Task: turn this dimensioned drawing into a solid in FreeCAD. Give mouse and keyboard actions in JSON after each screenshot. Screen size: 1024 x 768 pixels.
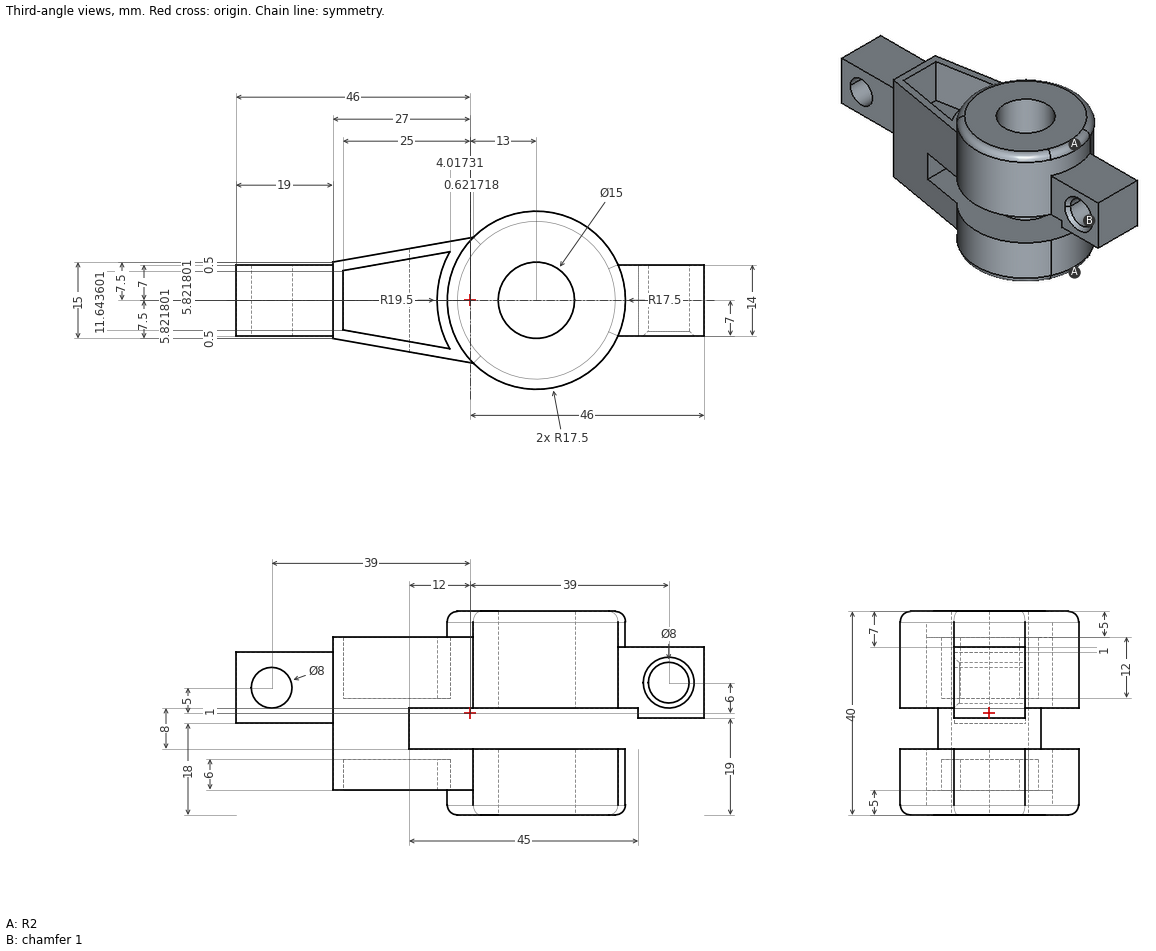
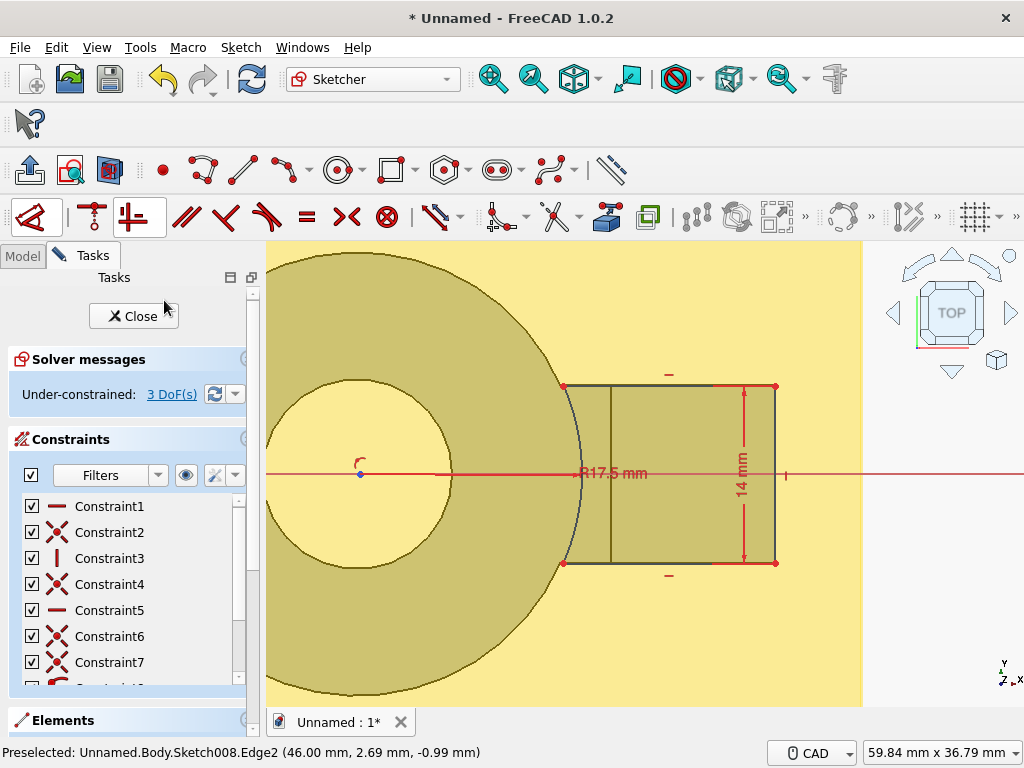
{"action": "left_click", "coordinate": [564, 386]}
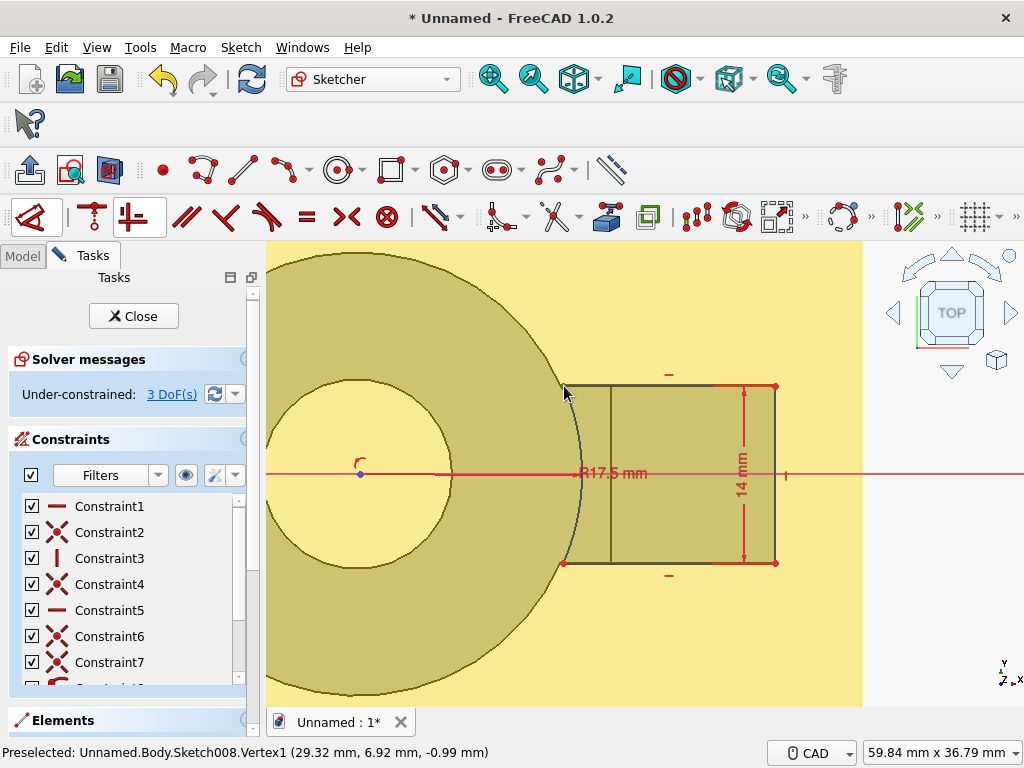
{"action": "left_click", "coordinate": [56, 218]}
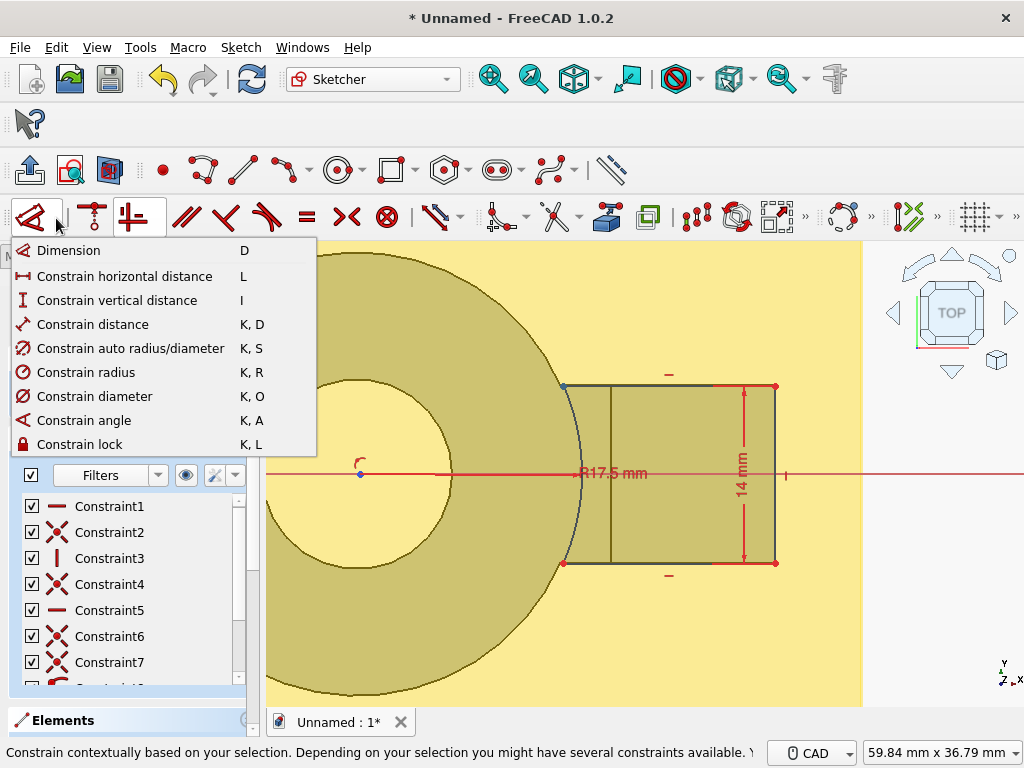
{"action": "left_click", "coordinate": [164, 300]}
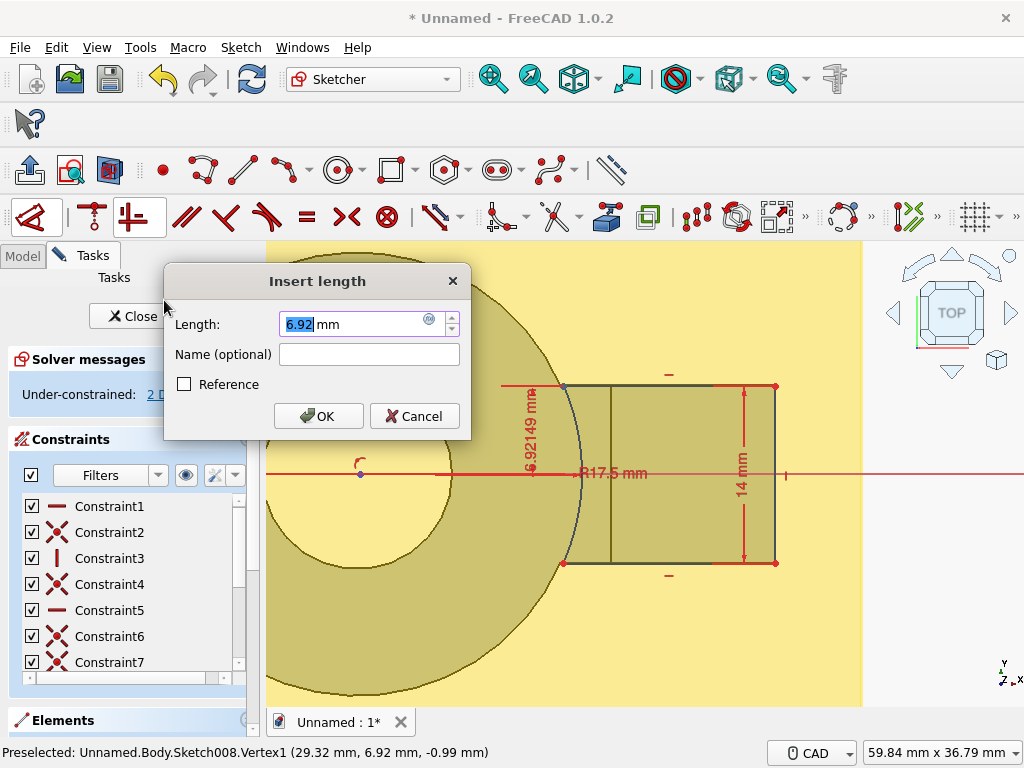
{"action": "type", "text": "7"}
{"action": "key", "text": "Return"}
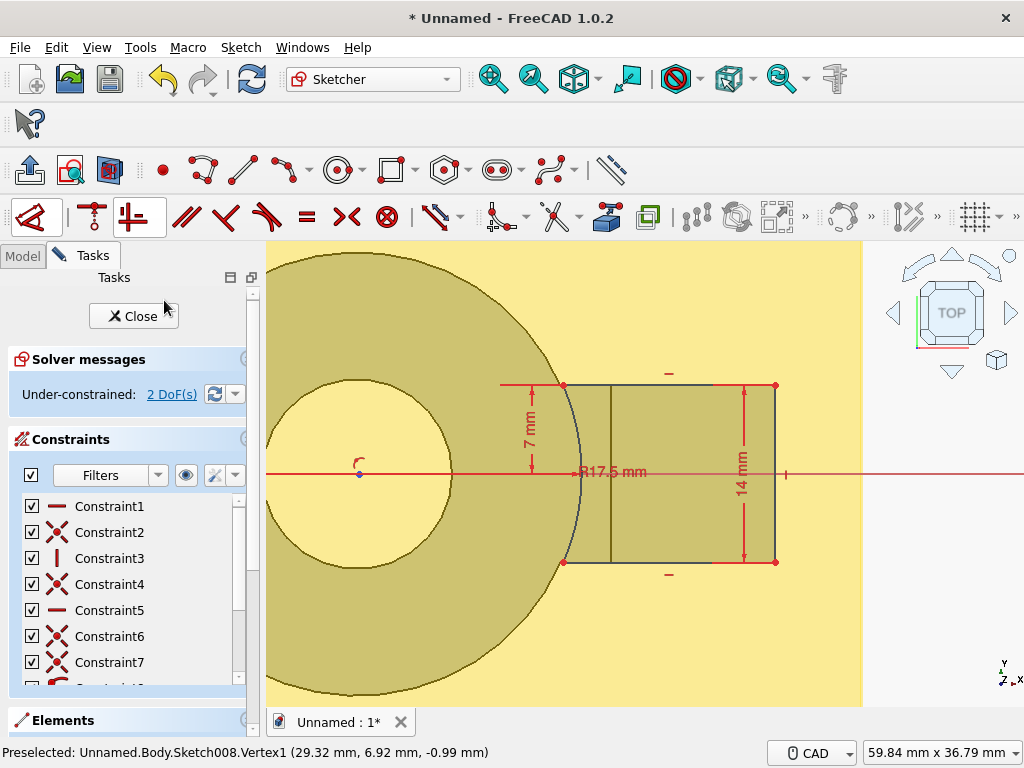
{"action": "left_click", "coordinate": [775, 385]}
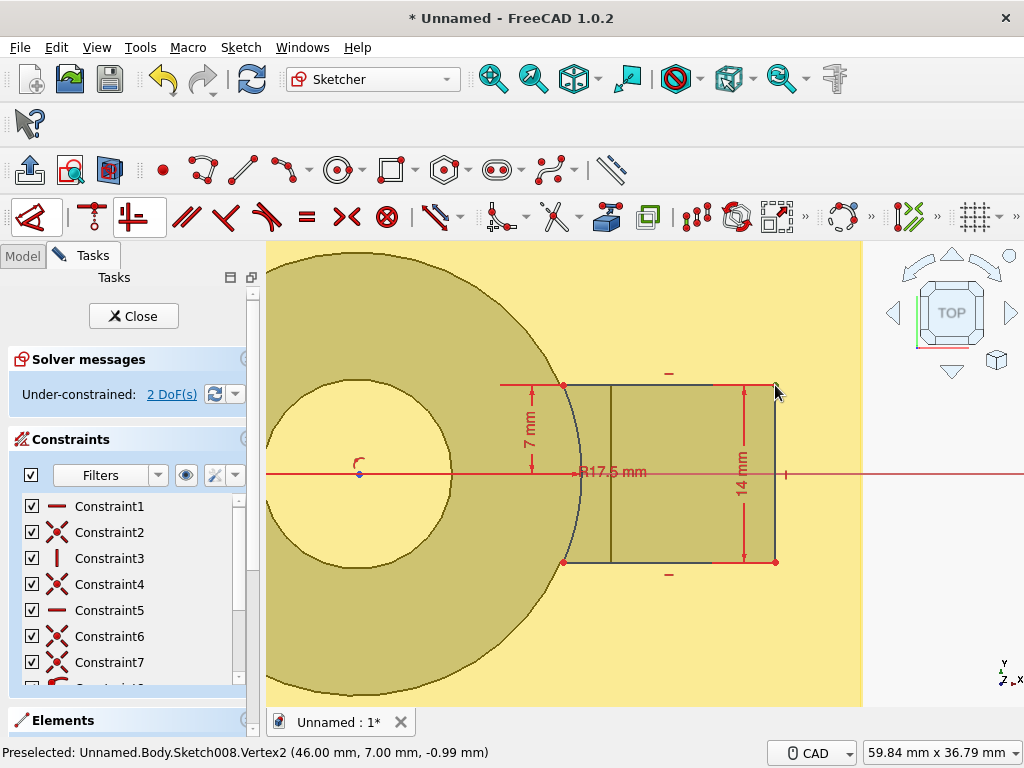
{"action": "left_click", "coordinate": [56, 218]}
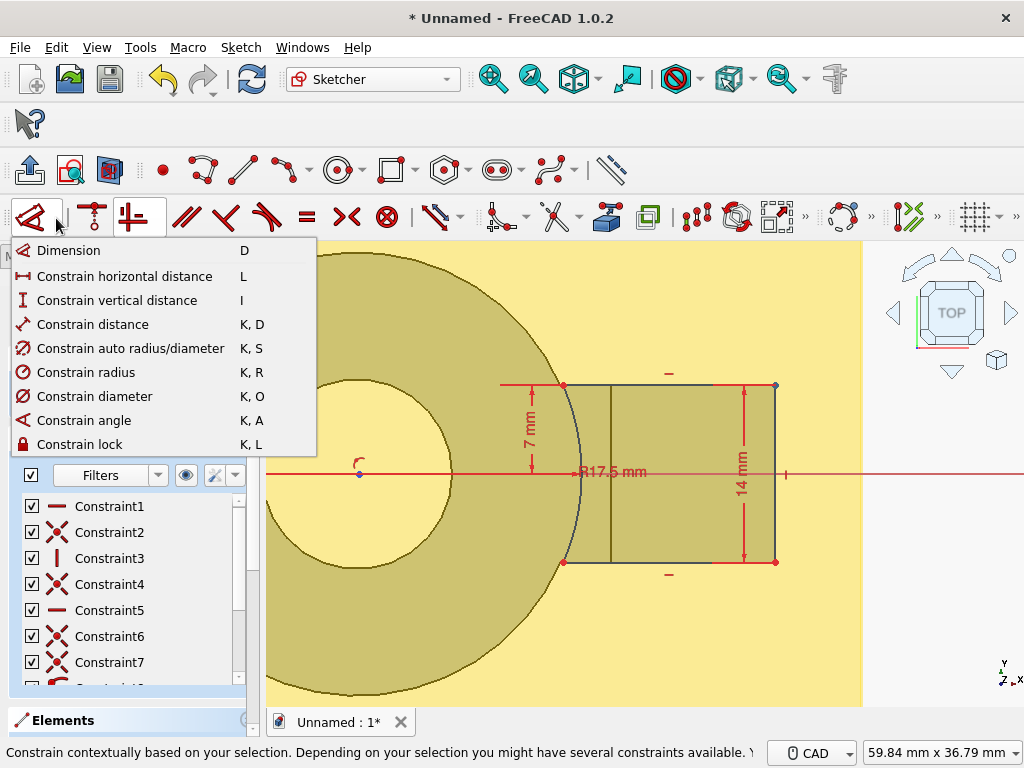
{"action": "left_click", "coordinate": [164, 276]}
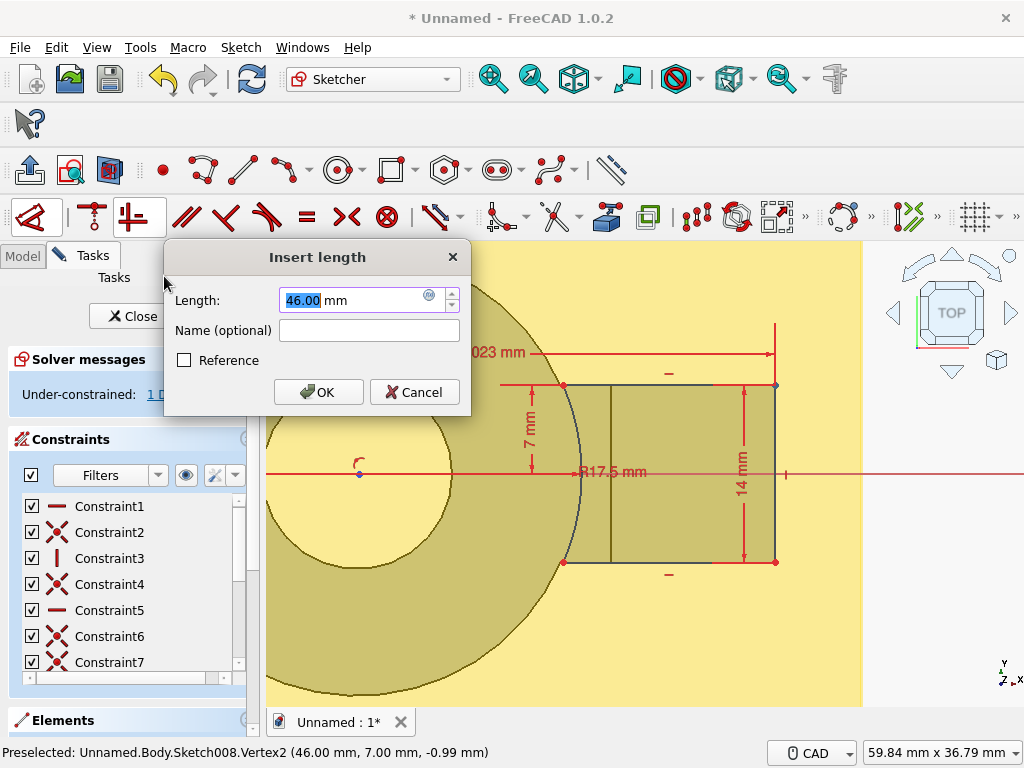
{"action": "type", "text": "46"}
{"action": "key", "text": "Return"}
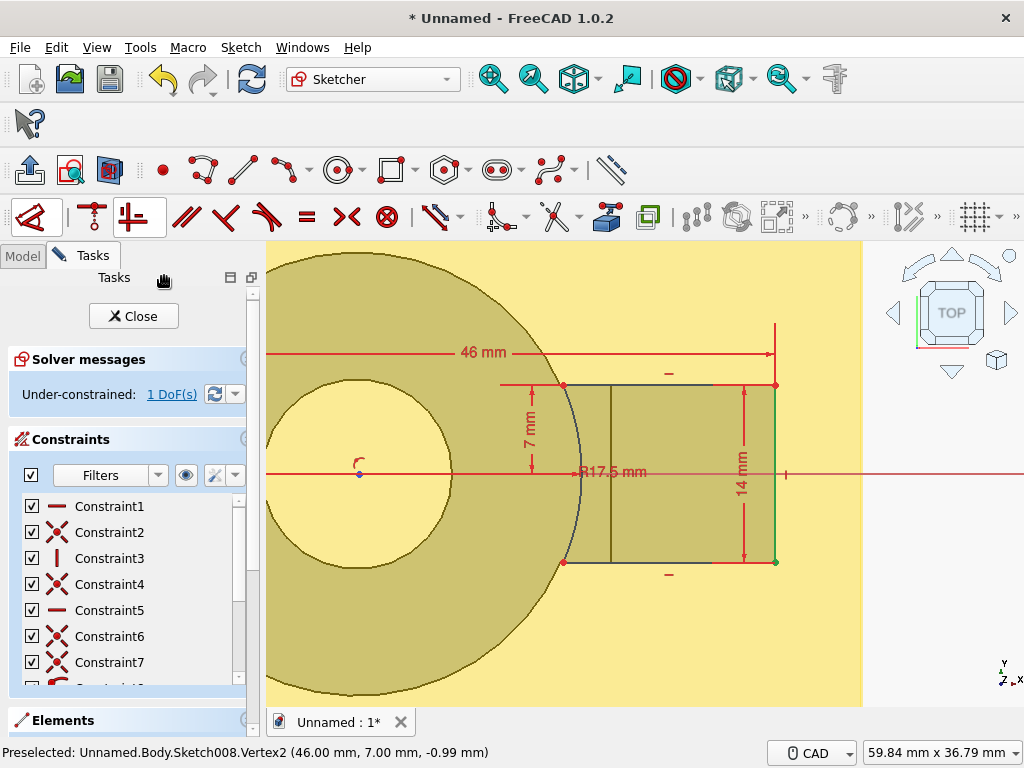
{"action": "left_click", "coordinate": [360, 474]}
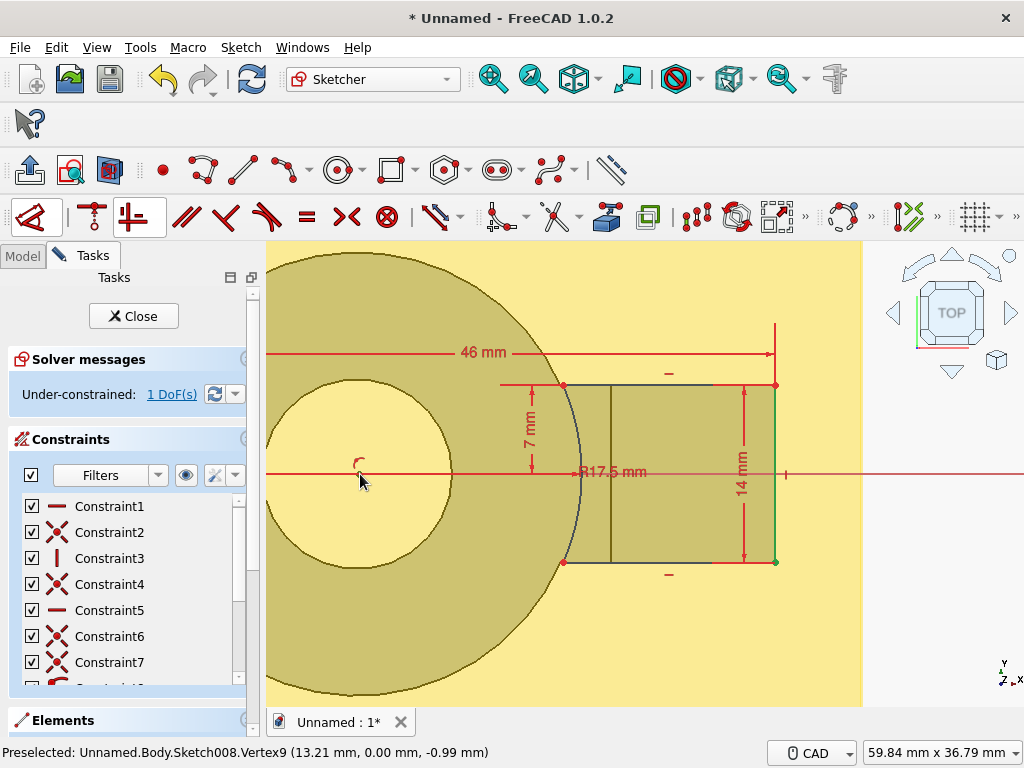
{"action": "key", "text": "l"}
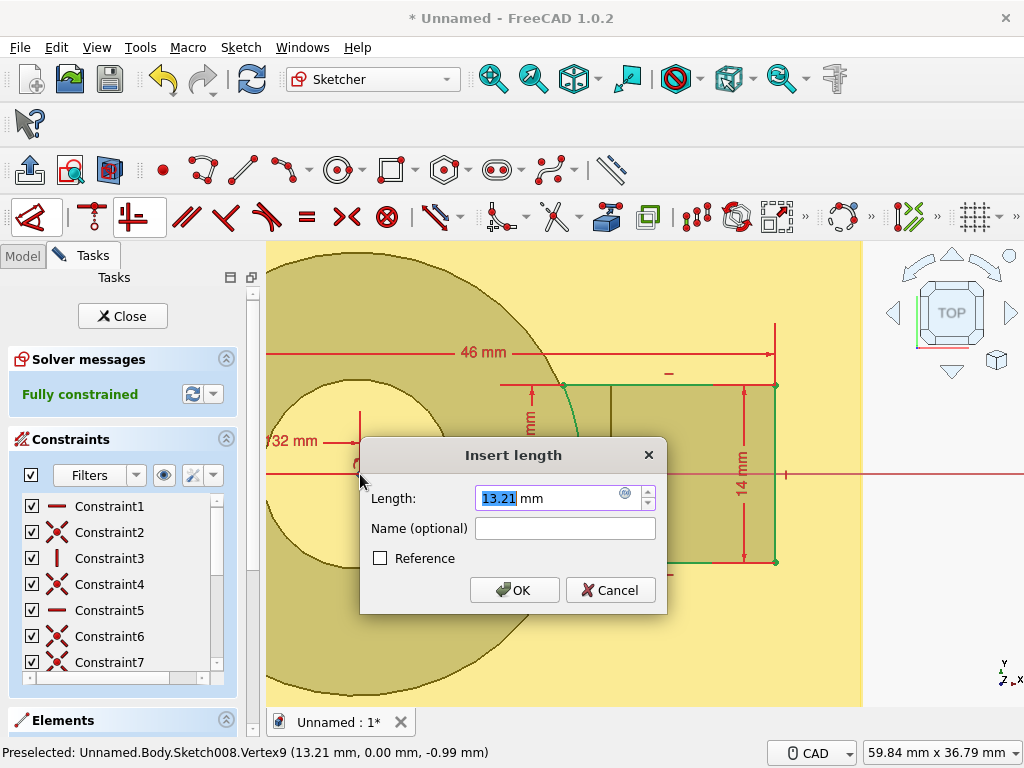
{"action": "type", "text": "13"}
{"action": "key", "text": "Return"}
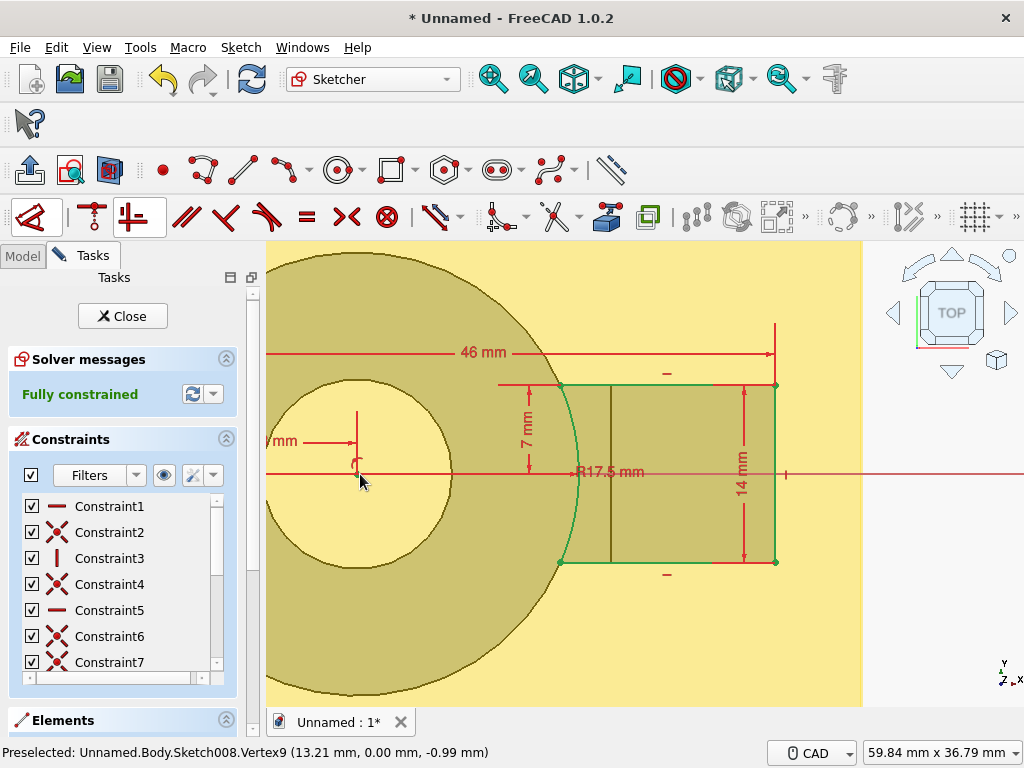
{"action": "left_click", "coordinate": [123, 316]}